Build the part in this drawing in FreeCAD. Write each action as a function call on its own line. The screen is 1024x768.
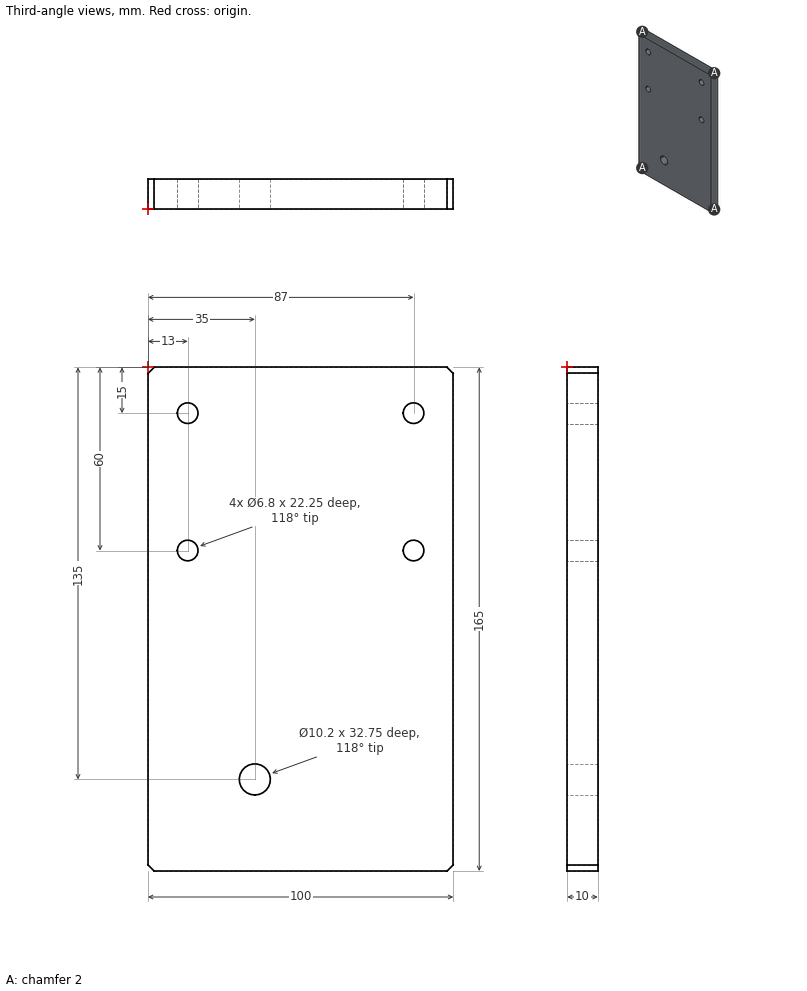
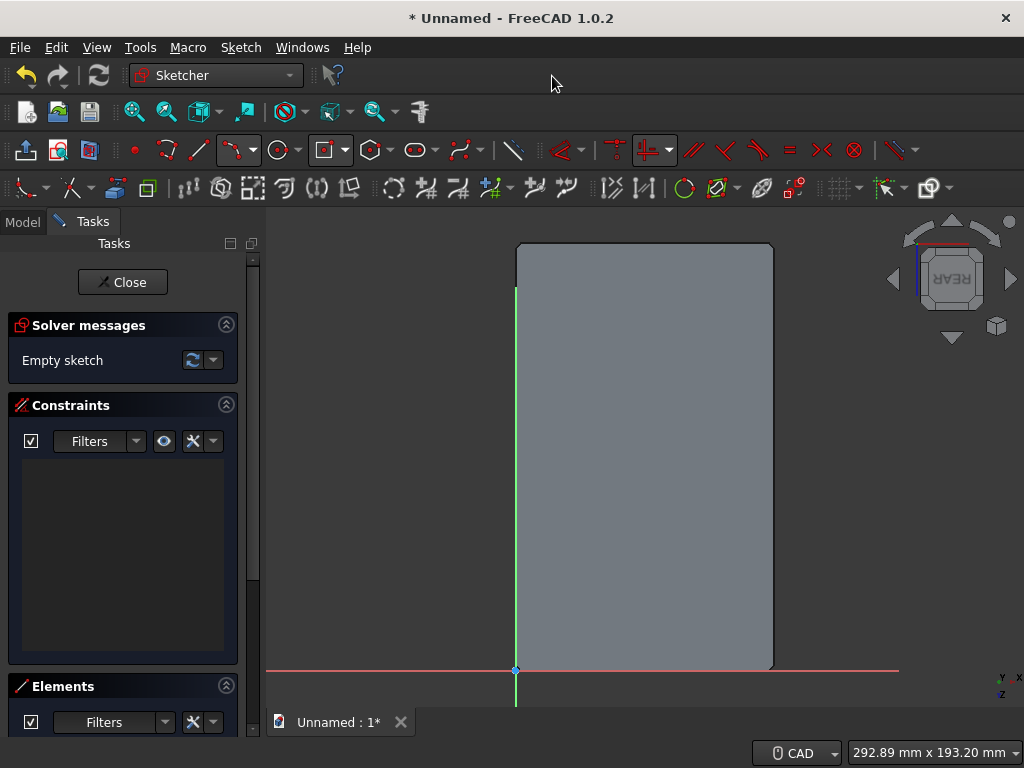
scroll(609, 308, up, 12)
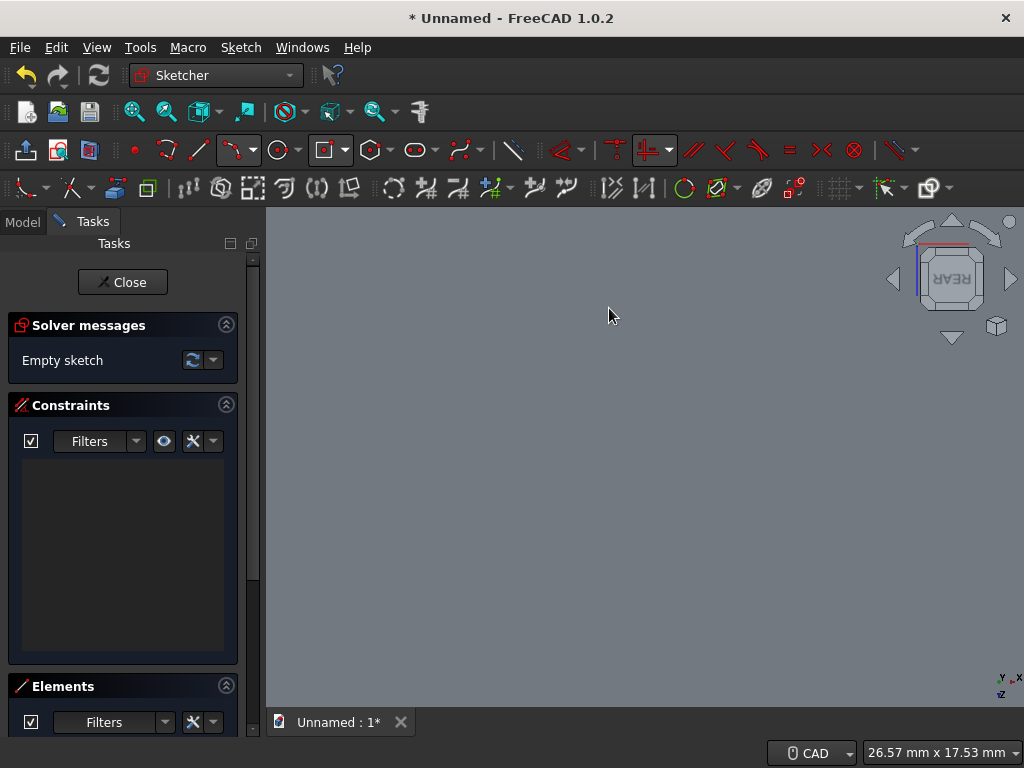
click(278, 150)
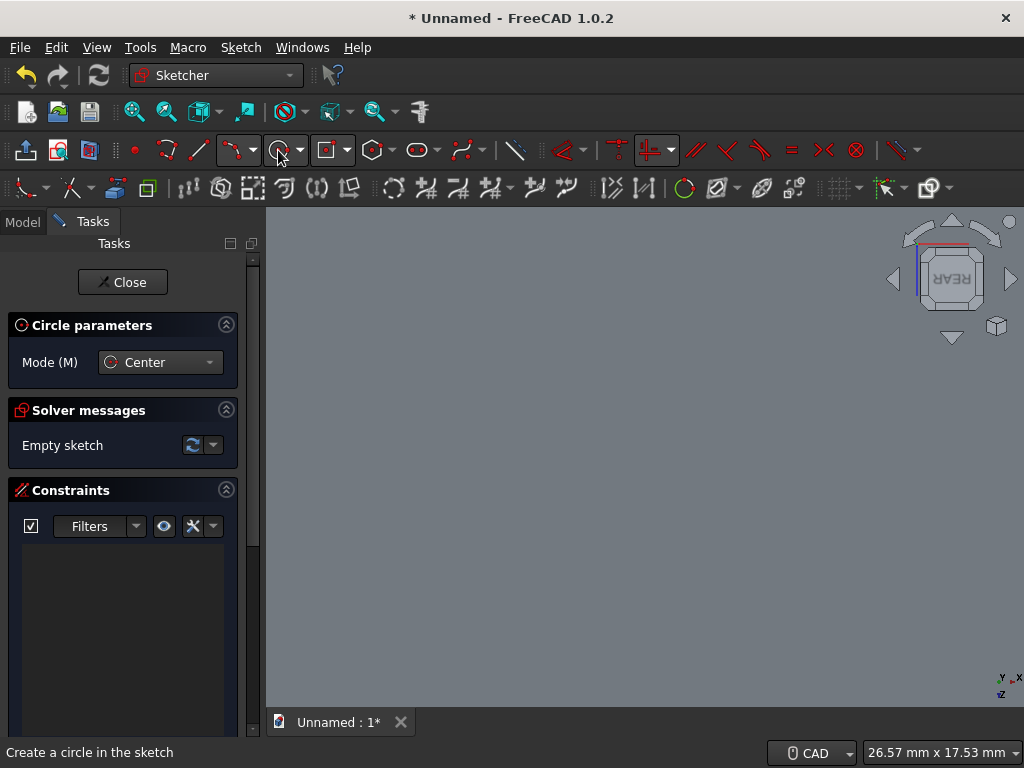
click(573, 451)
move(676, 348)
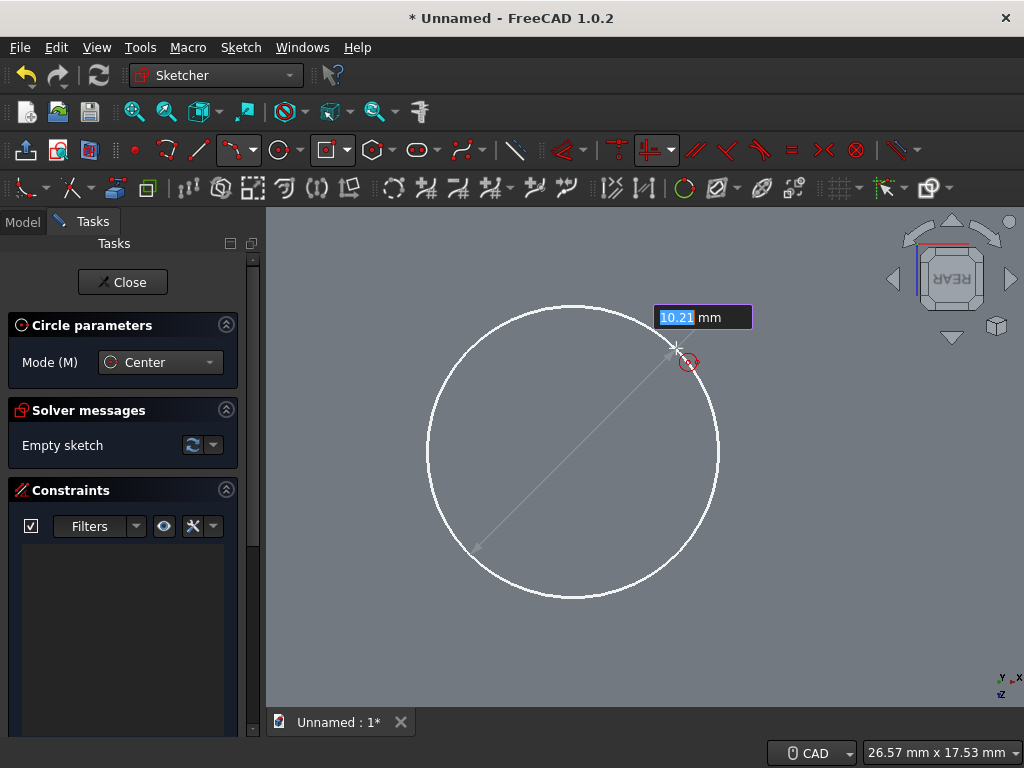
text(10.2)
key(Return)
key(Escape)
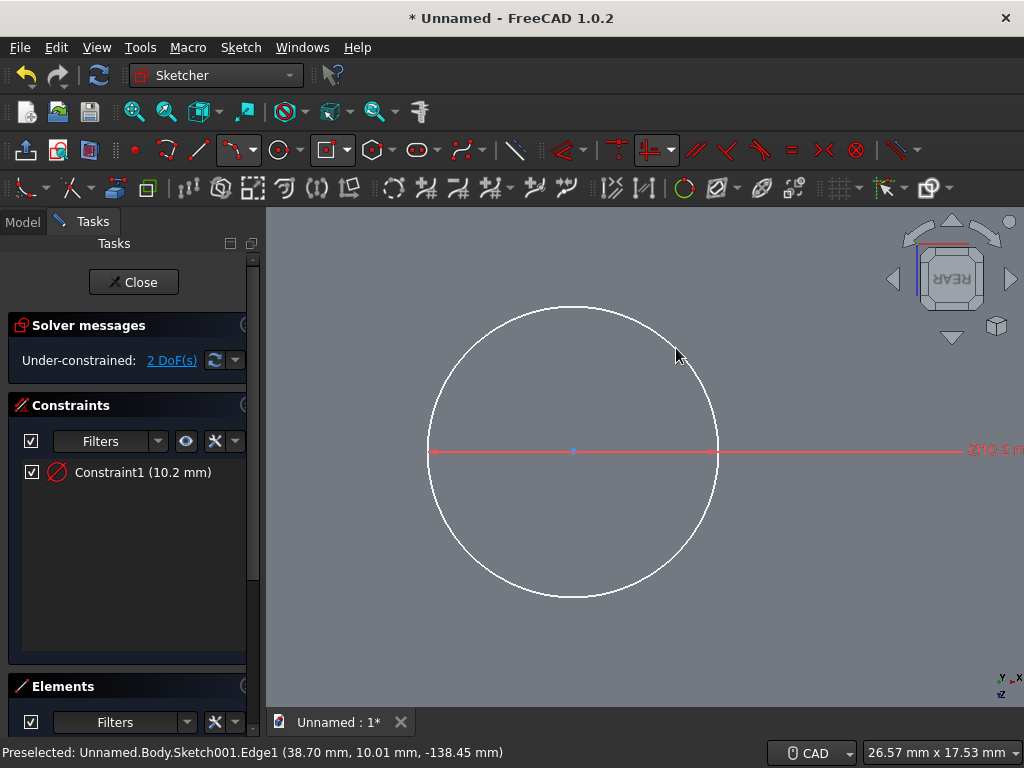
click(573, 452)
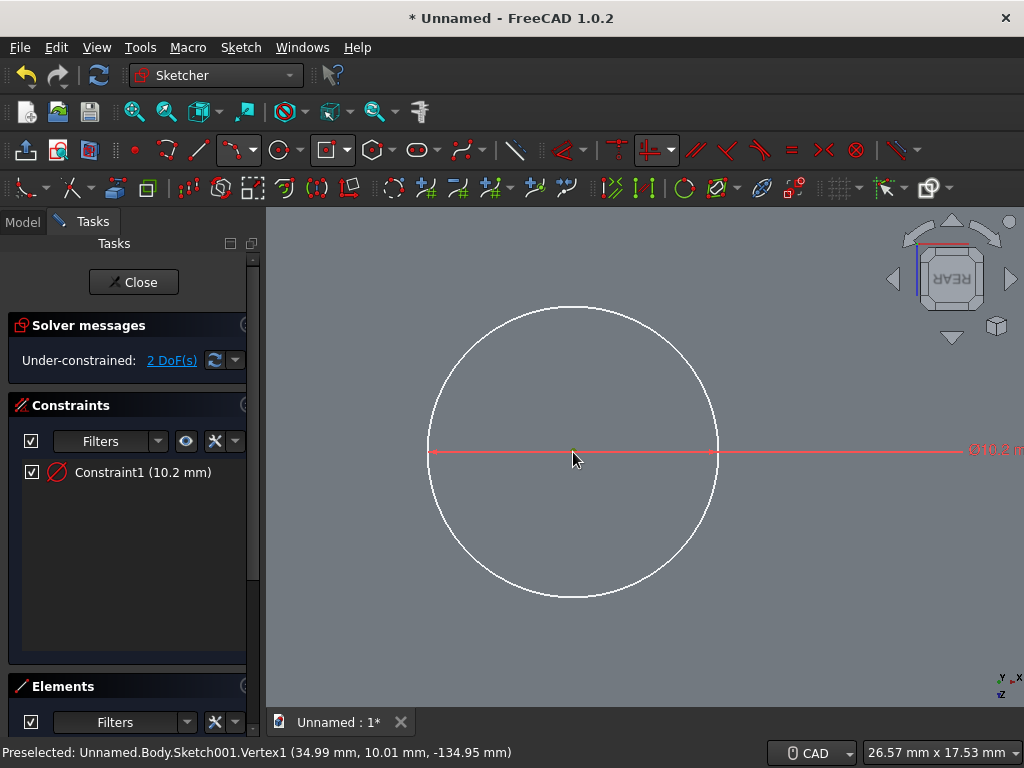
key(l)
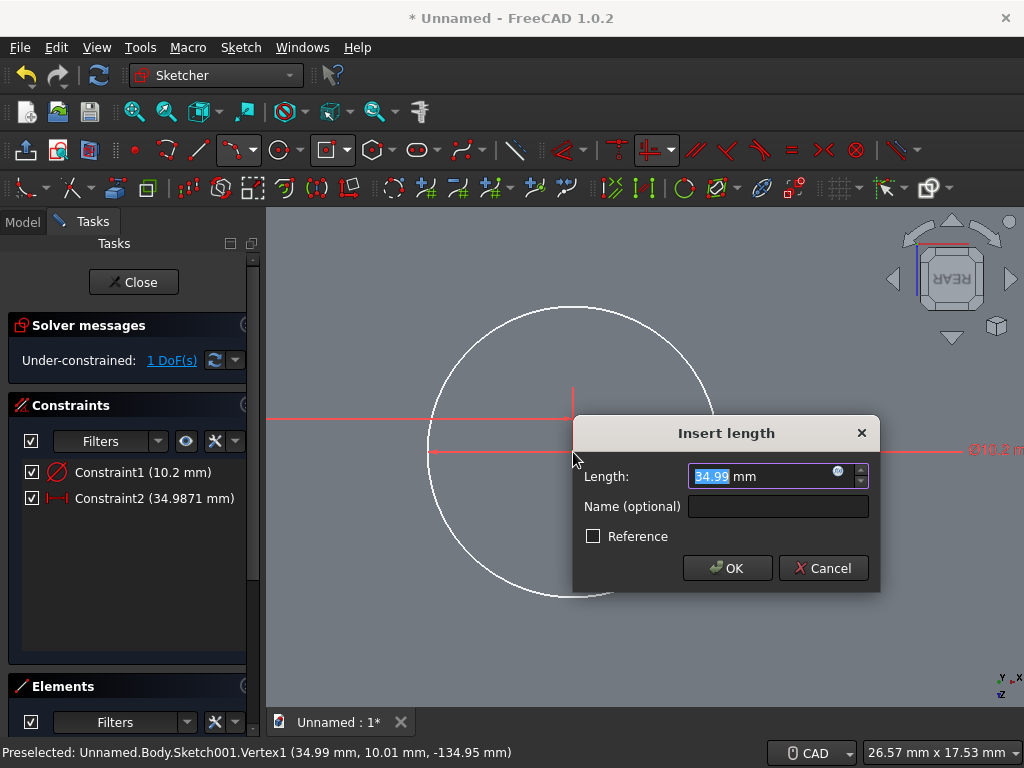
text(35)
key(Return)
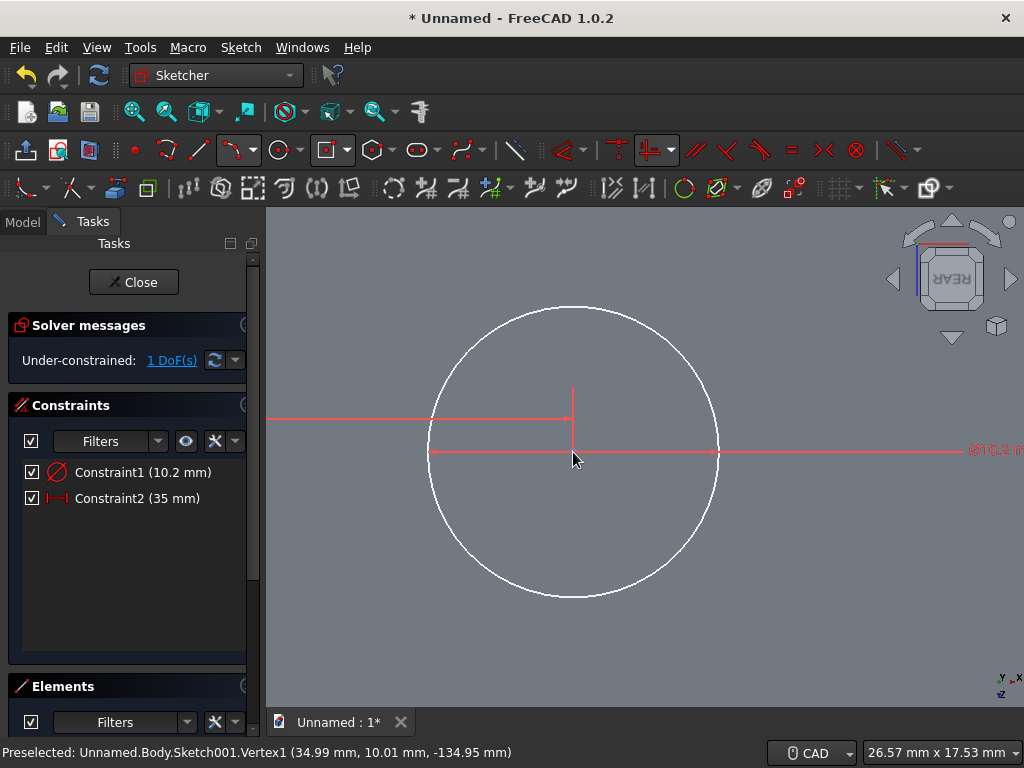
click(573, 452)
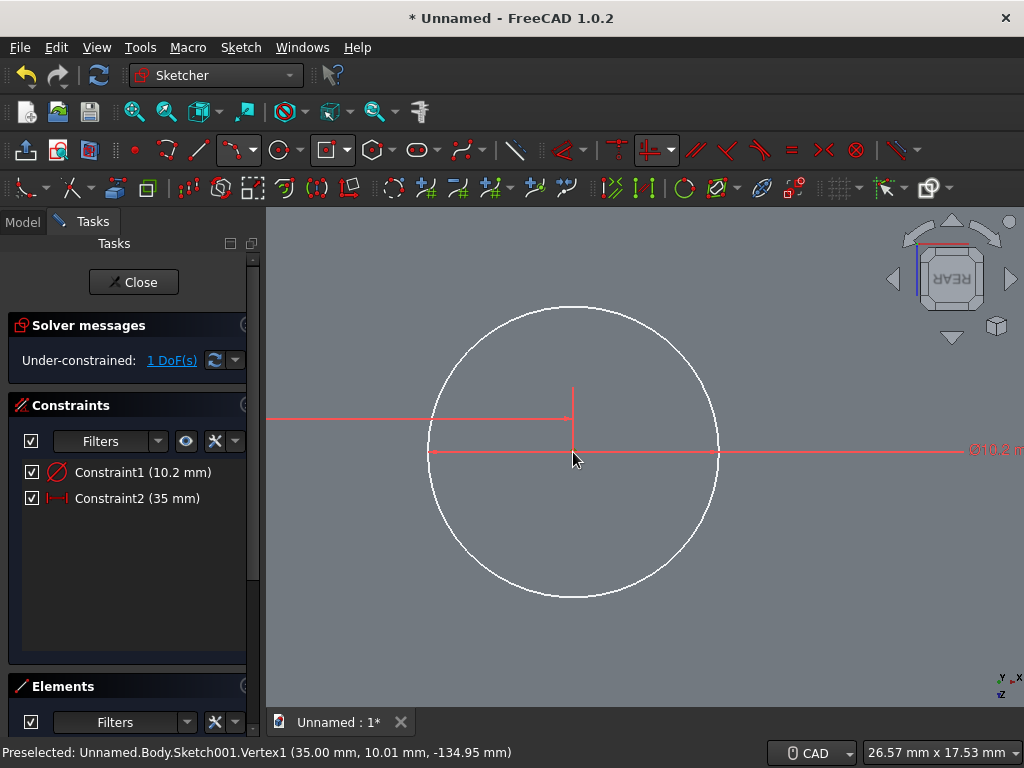
key(i)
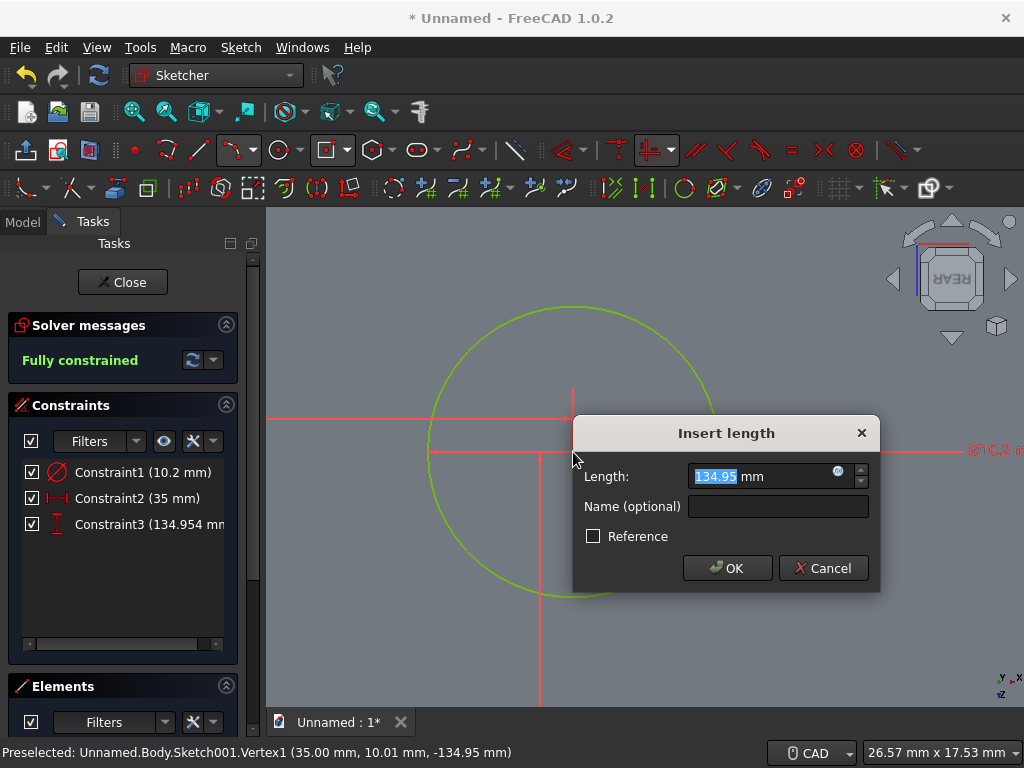
text(135)
key(Return)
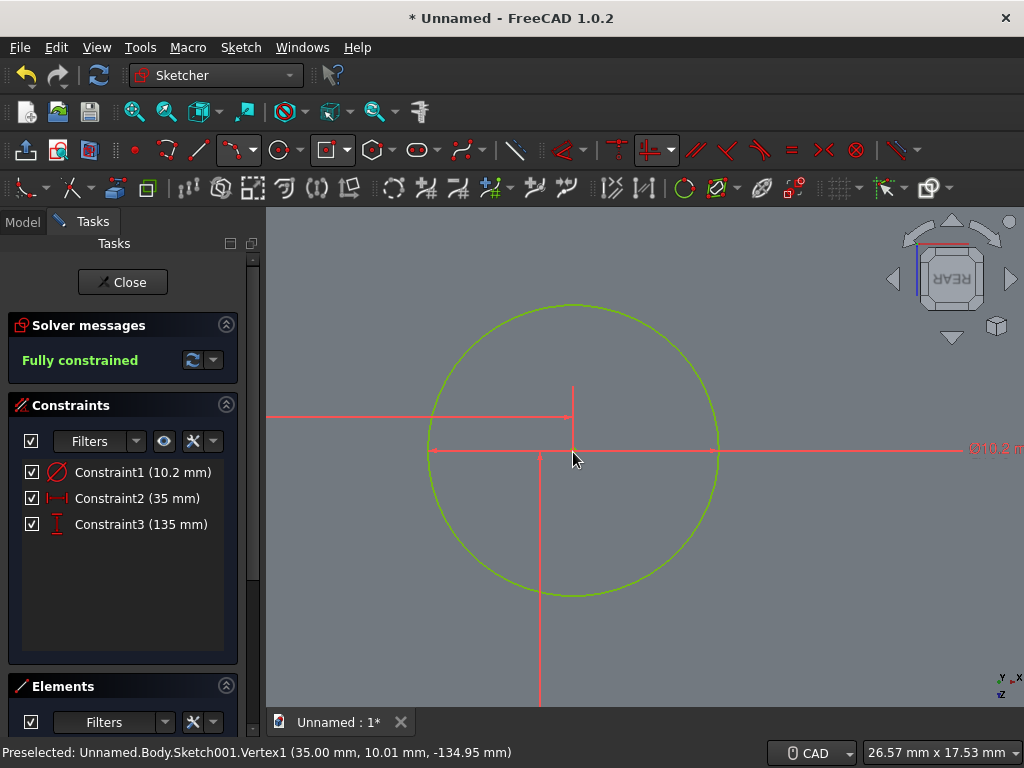
click(123, 282)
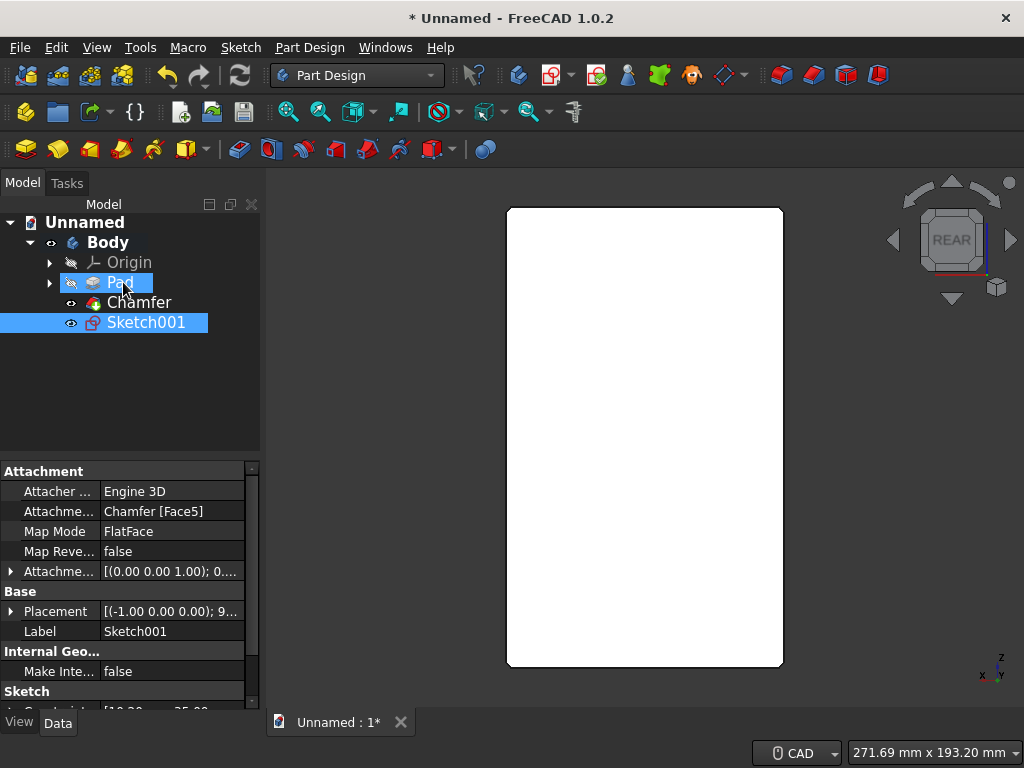
click(272, 150)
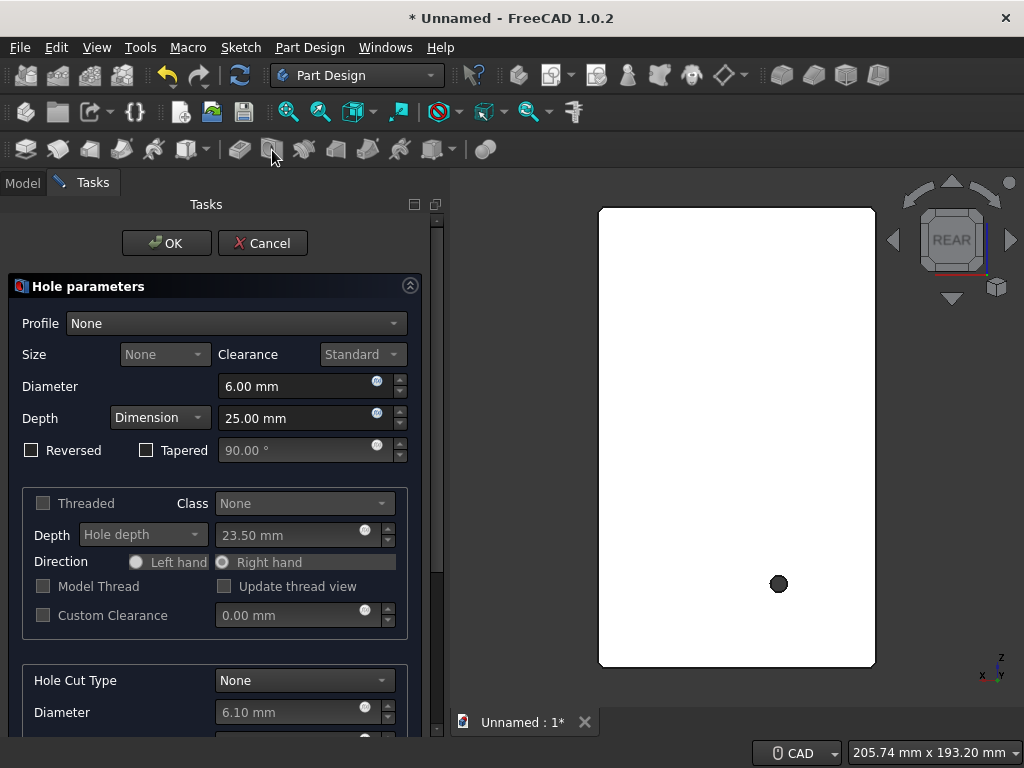
triple_click(305, 386)